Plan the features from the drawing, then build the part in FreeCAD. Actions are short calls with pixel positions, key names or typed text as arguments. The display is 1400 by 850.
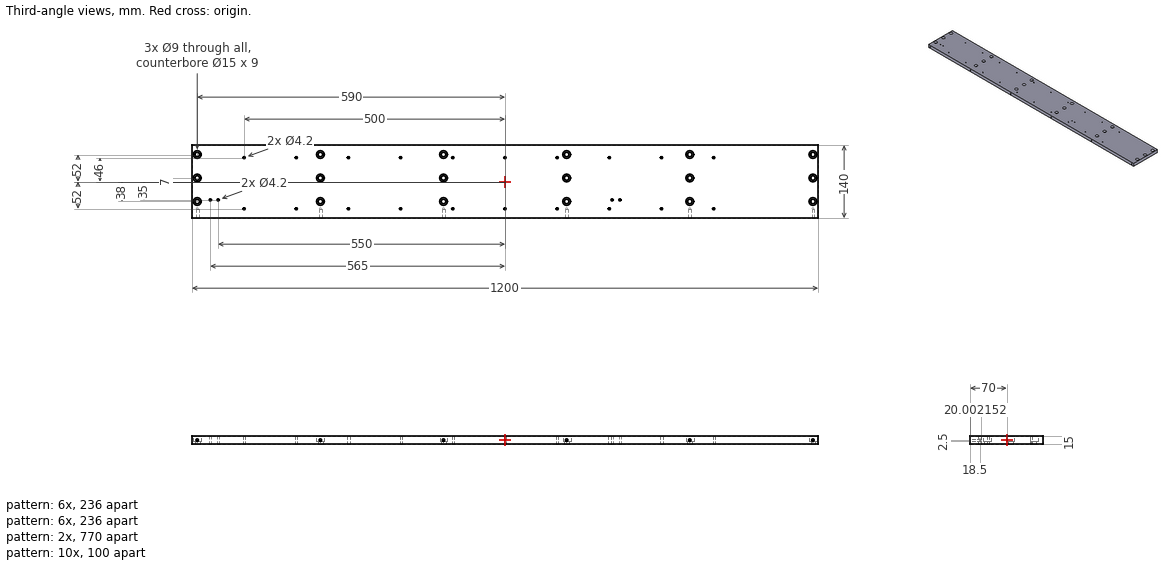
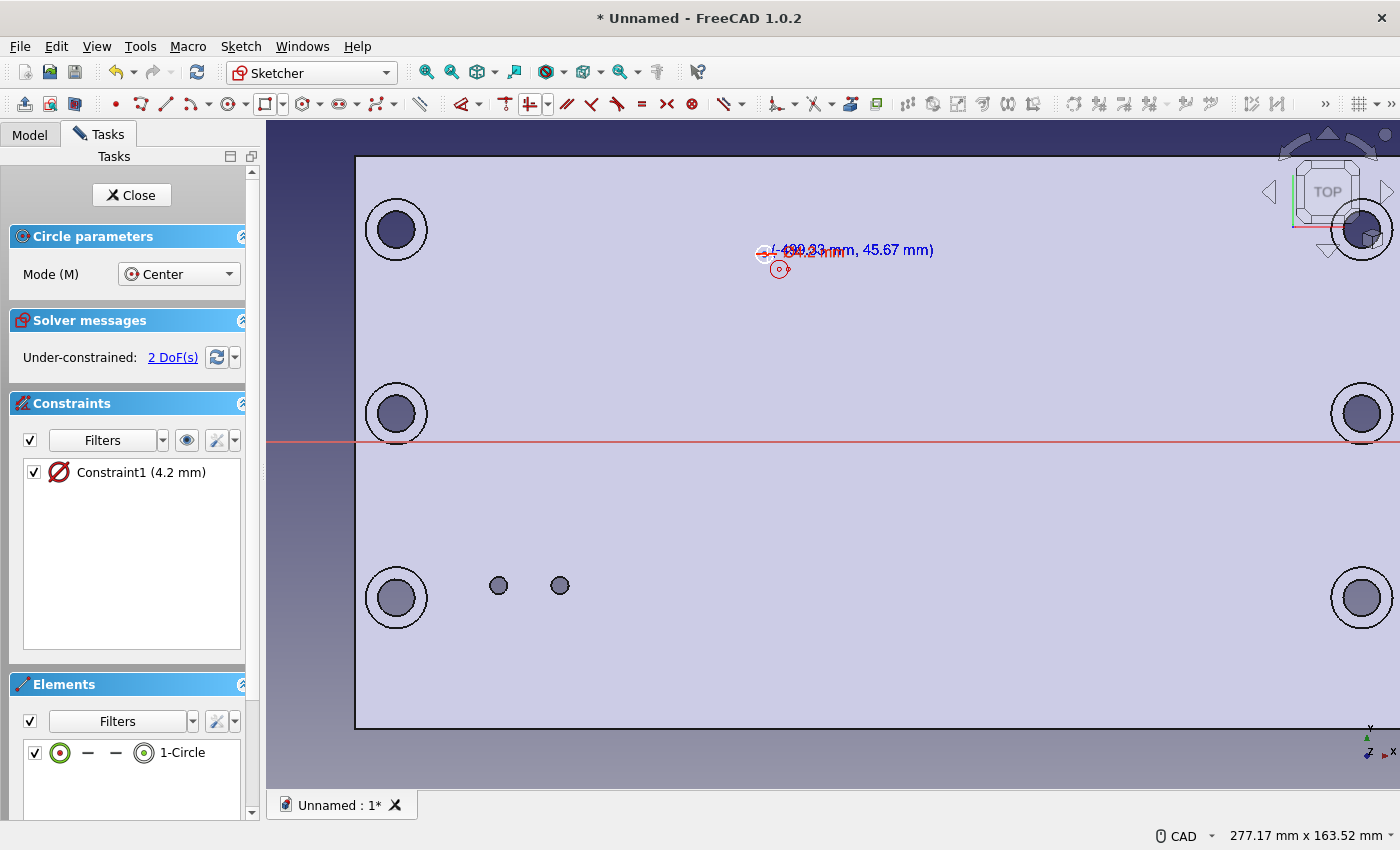
scroll(765, 655, up, 5)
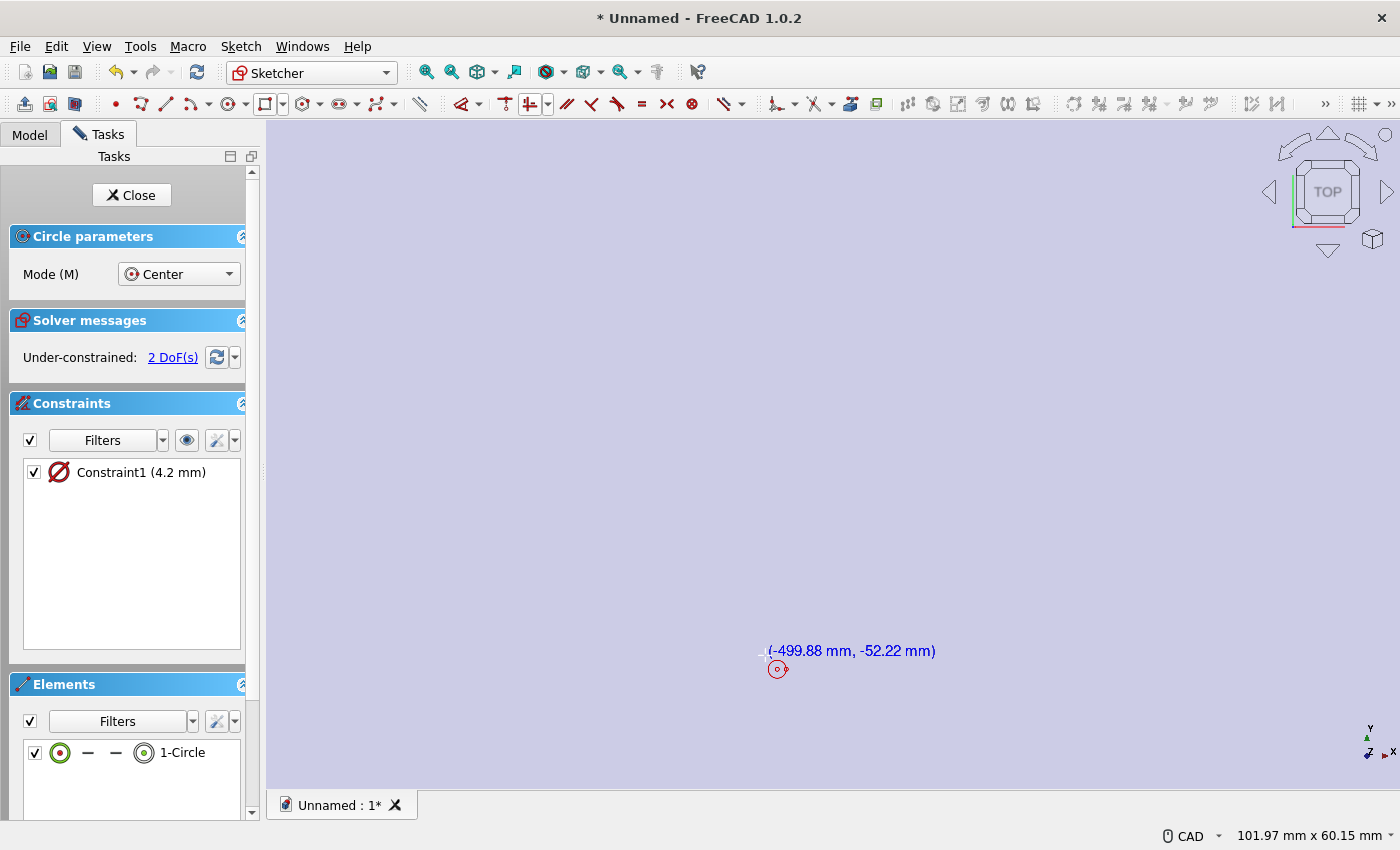
click(763, 654)
move(779, 637)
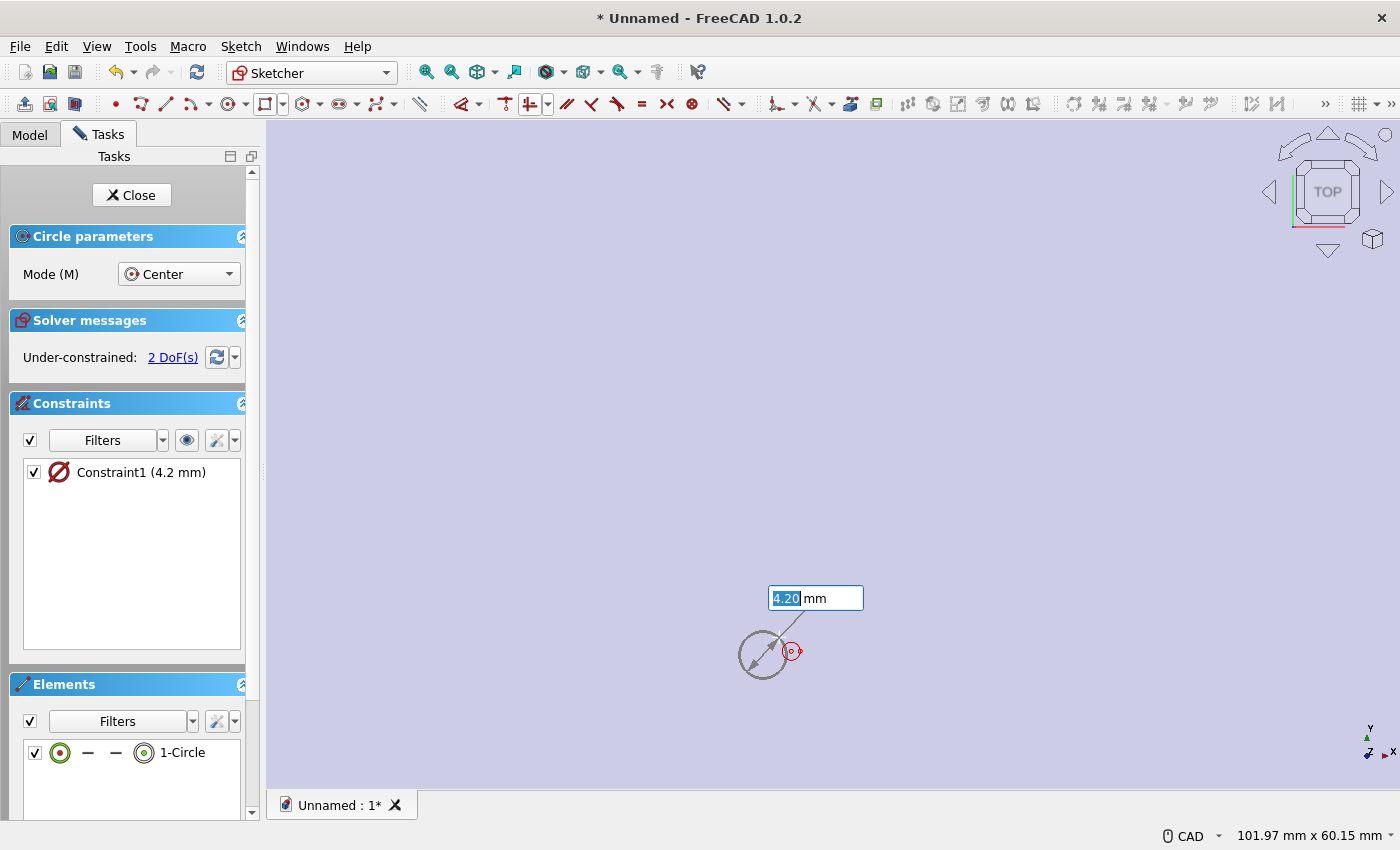
text(4.2)
key(Return)
key(Escape)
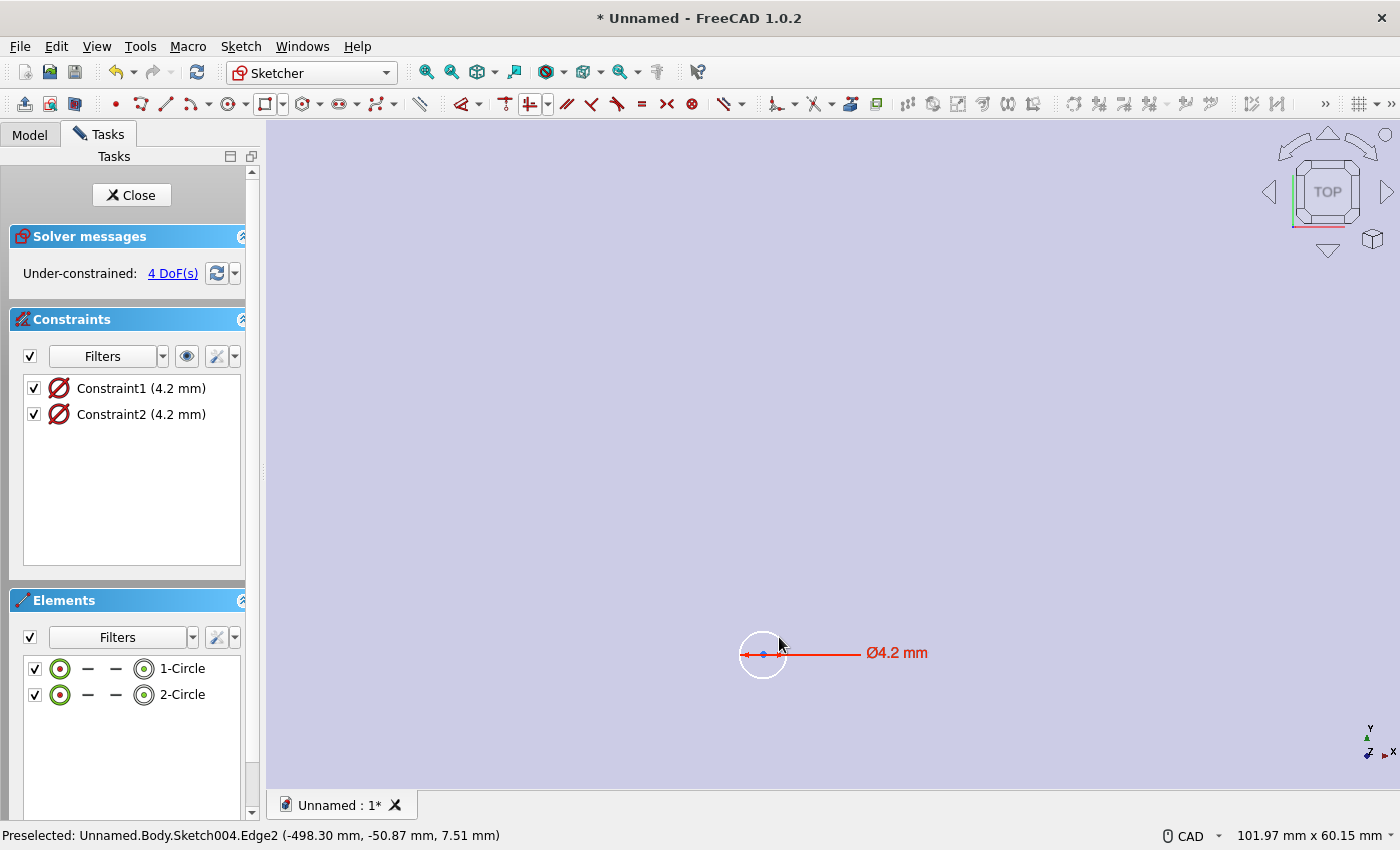
scroll(765, 656, down, 5)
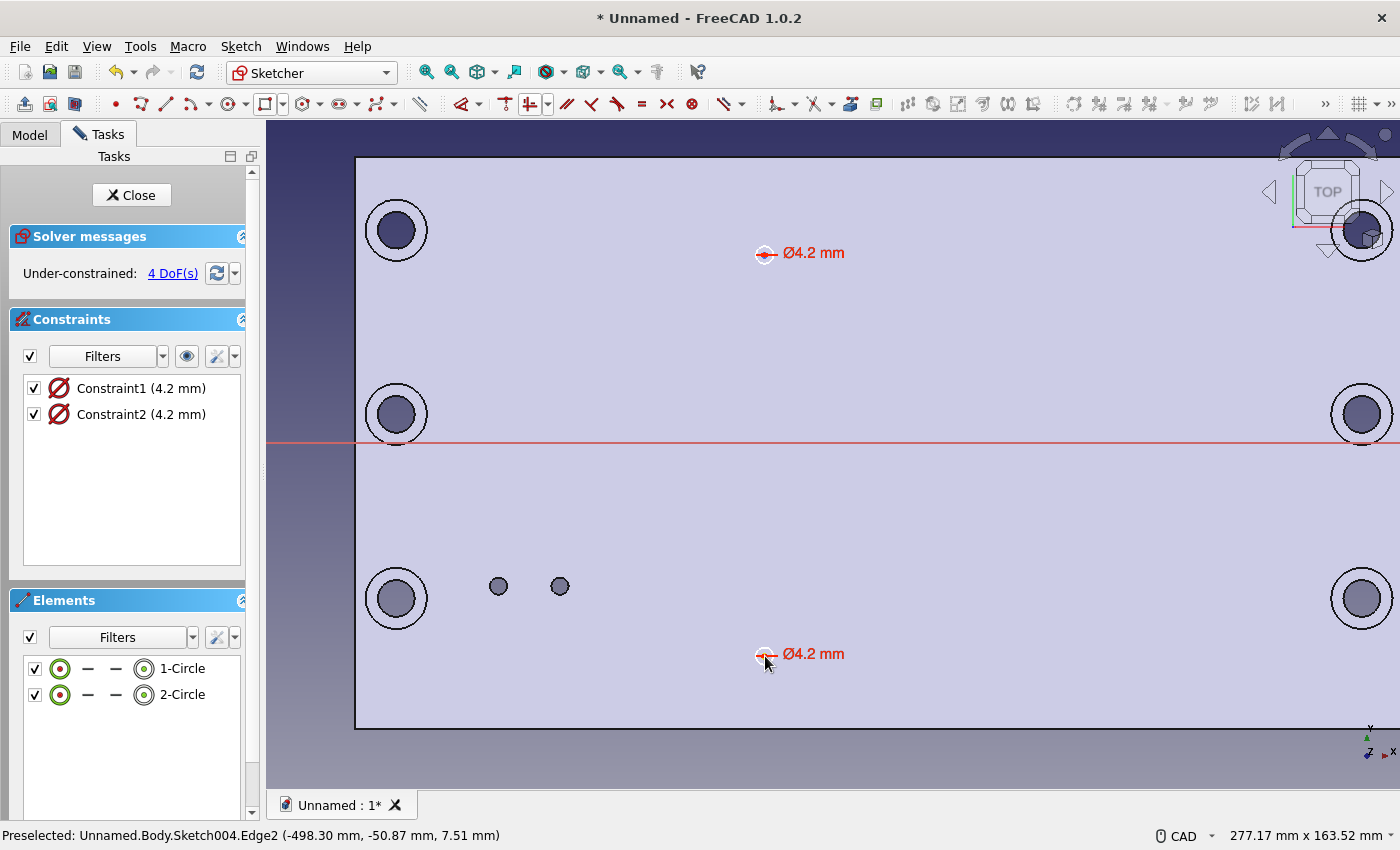
click(765, 255)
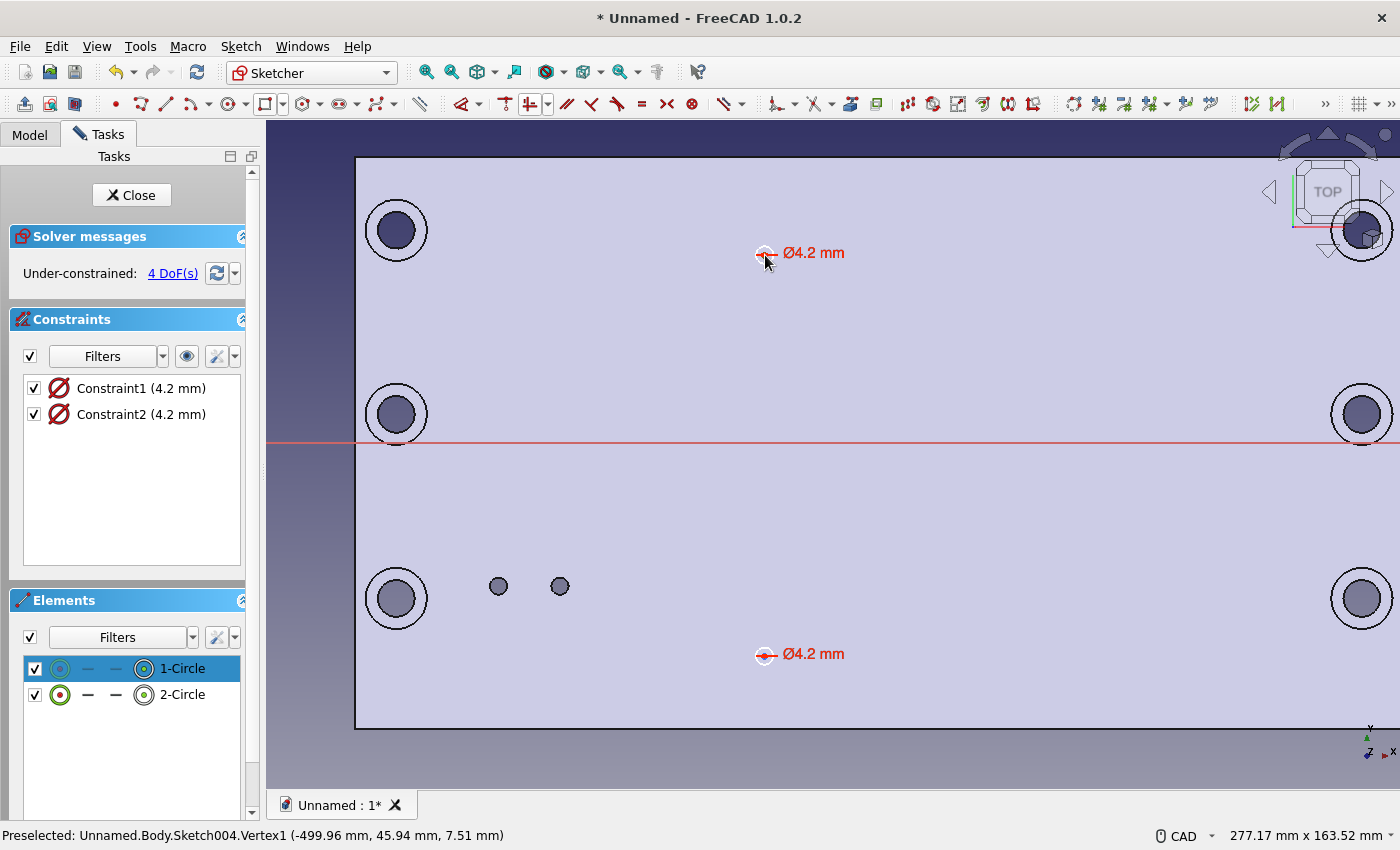
click(765, 656)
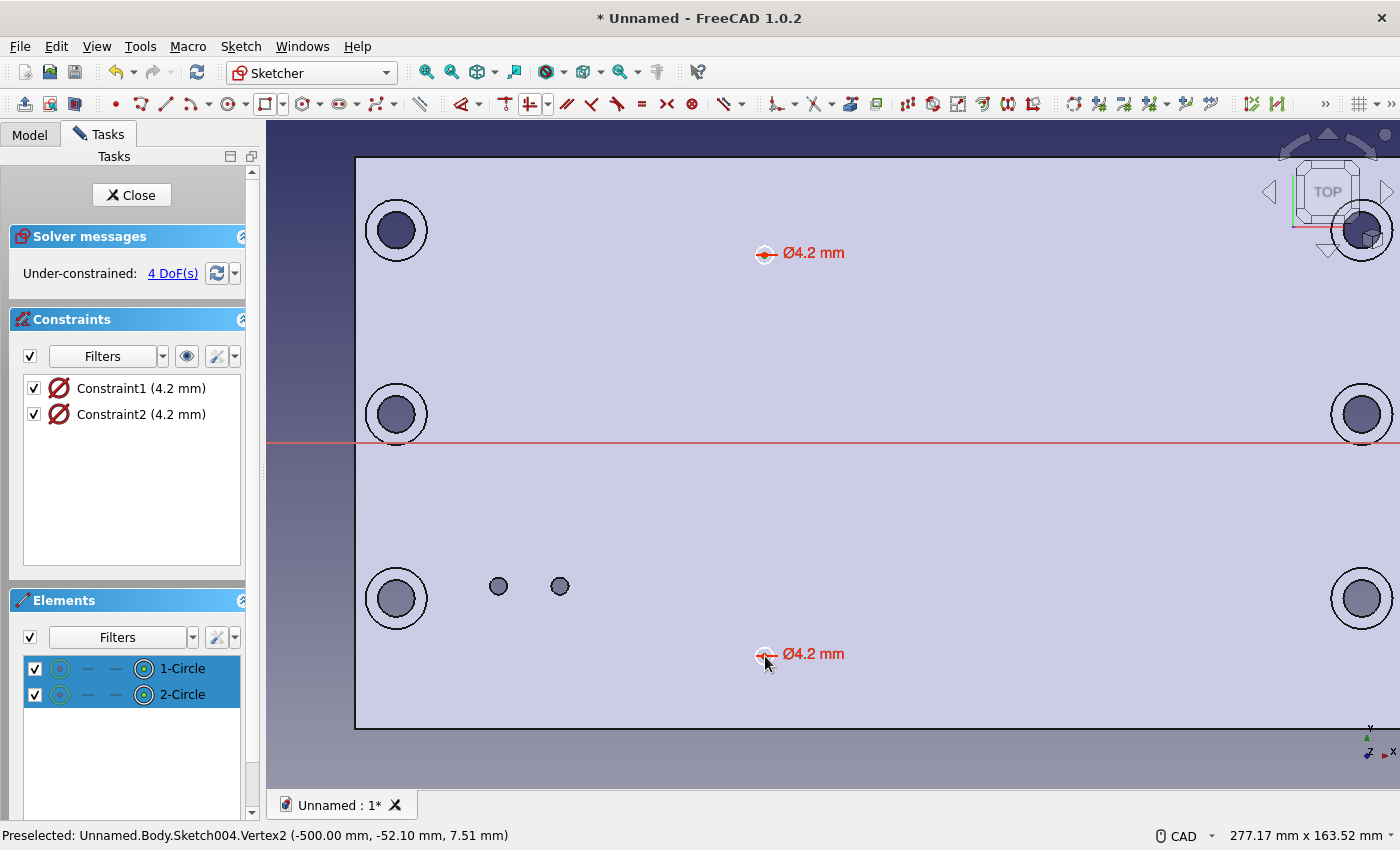
key(v)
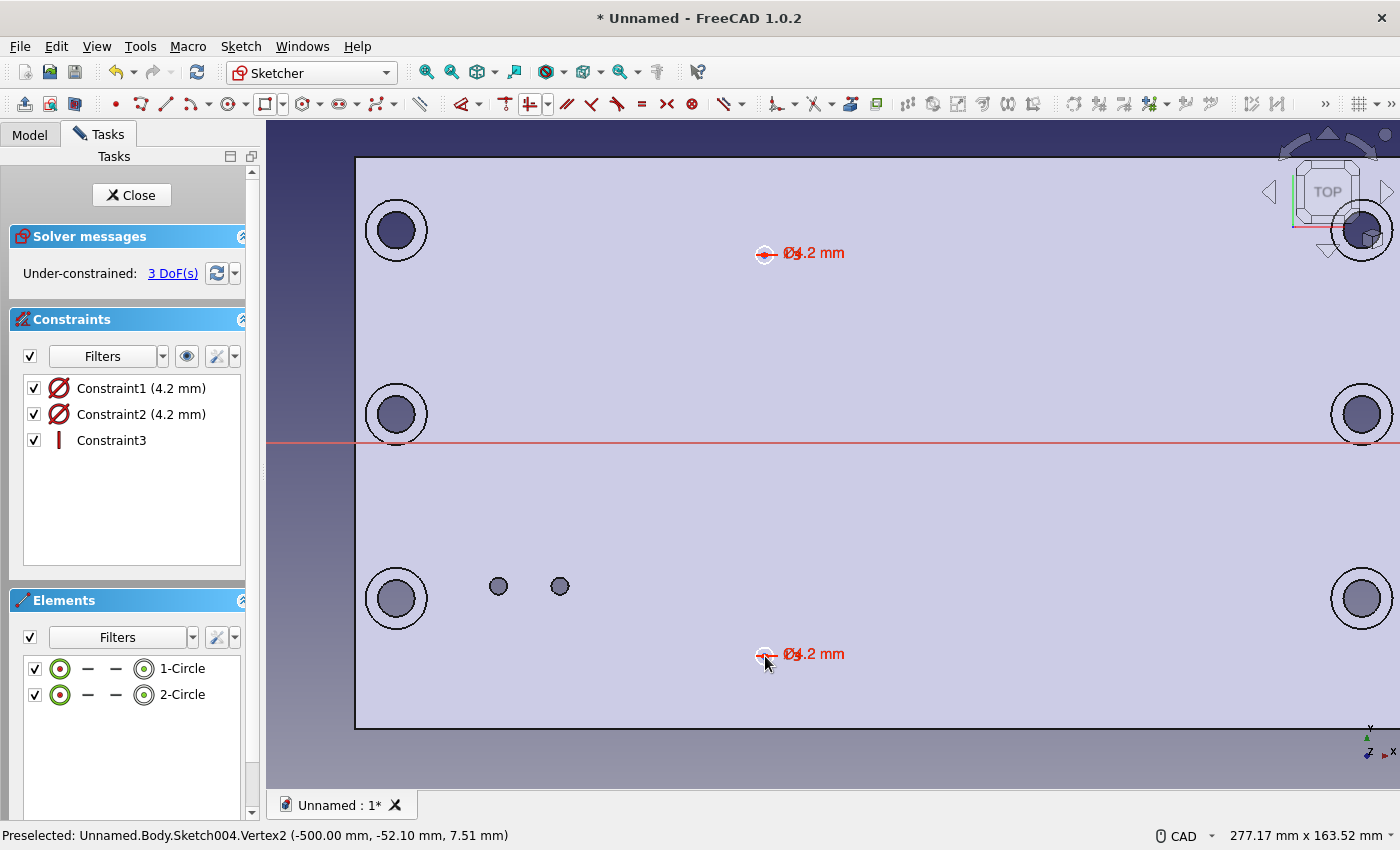
click(460, 104)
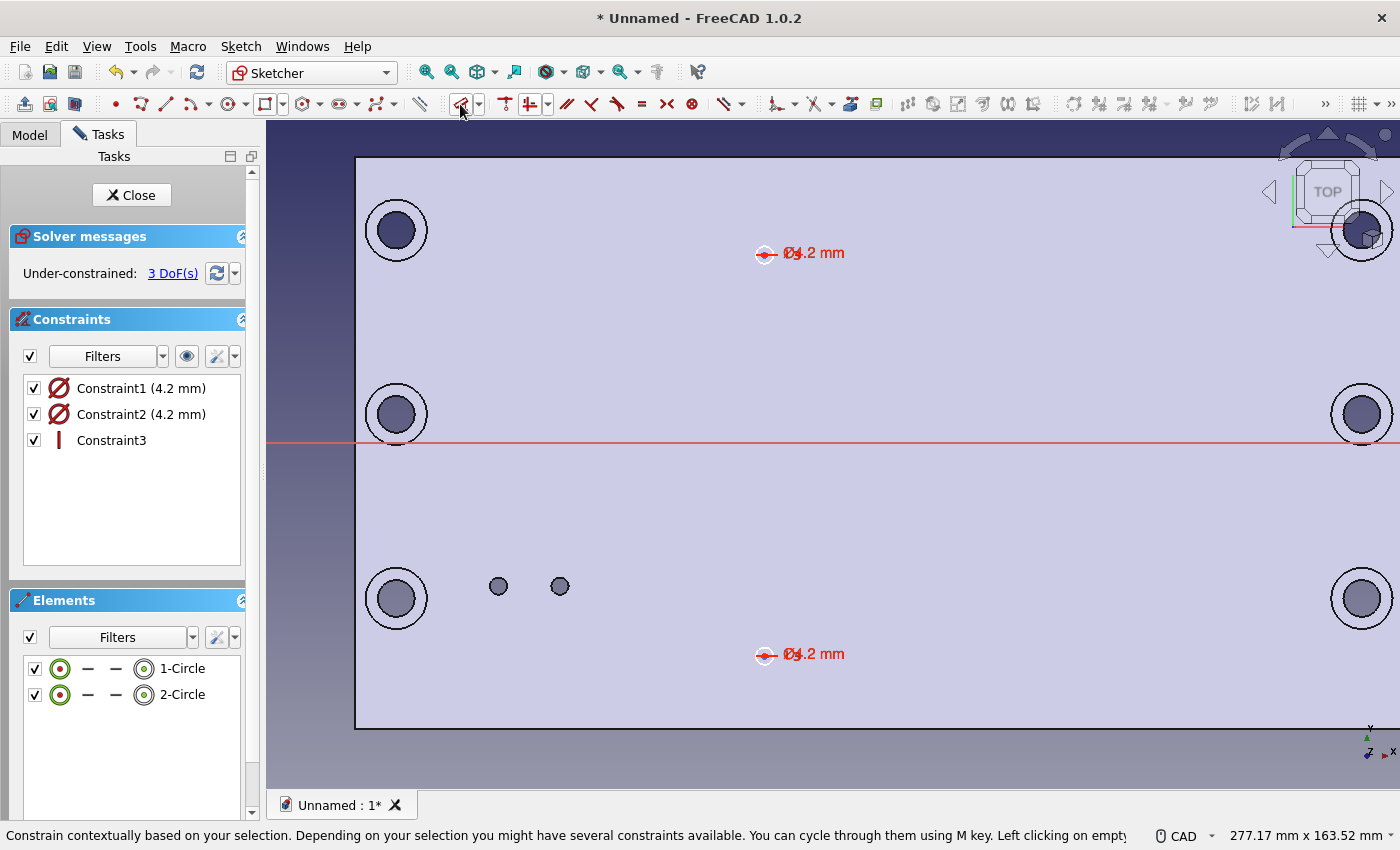
click(765, 255)
click(731, 349)